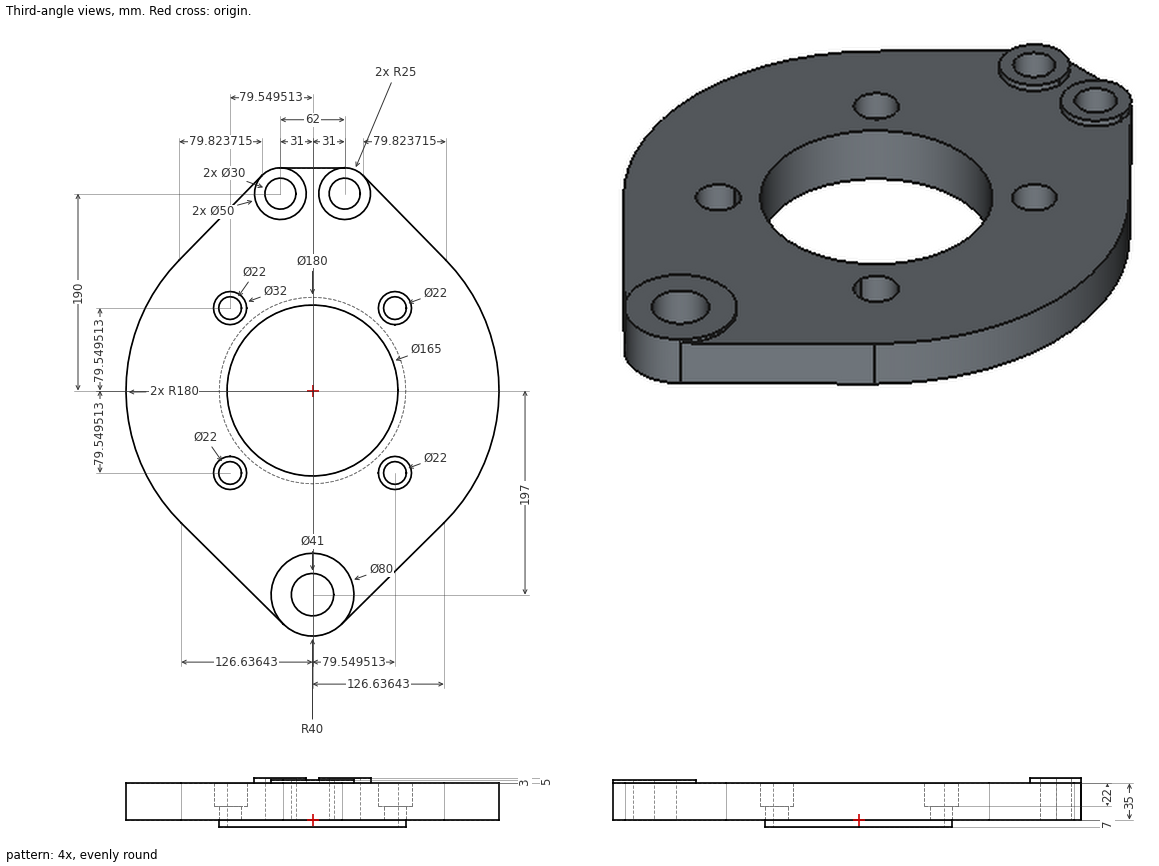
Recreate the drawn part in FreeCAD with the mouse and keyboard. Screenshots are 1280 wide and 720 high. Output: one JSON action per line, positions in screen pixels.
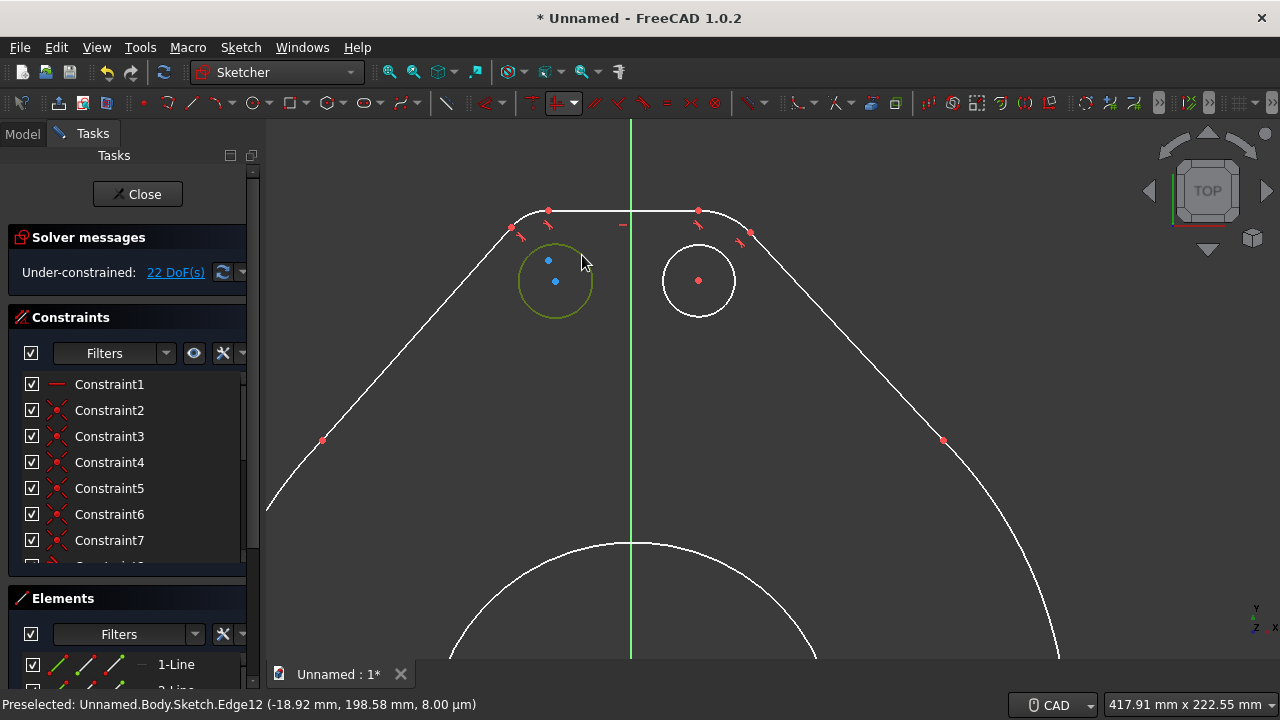
{"action": "left_click", "coordinate": [536, 212]}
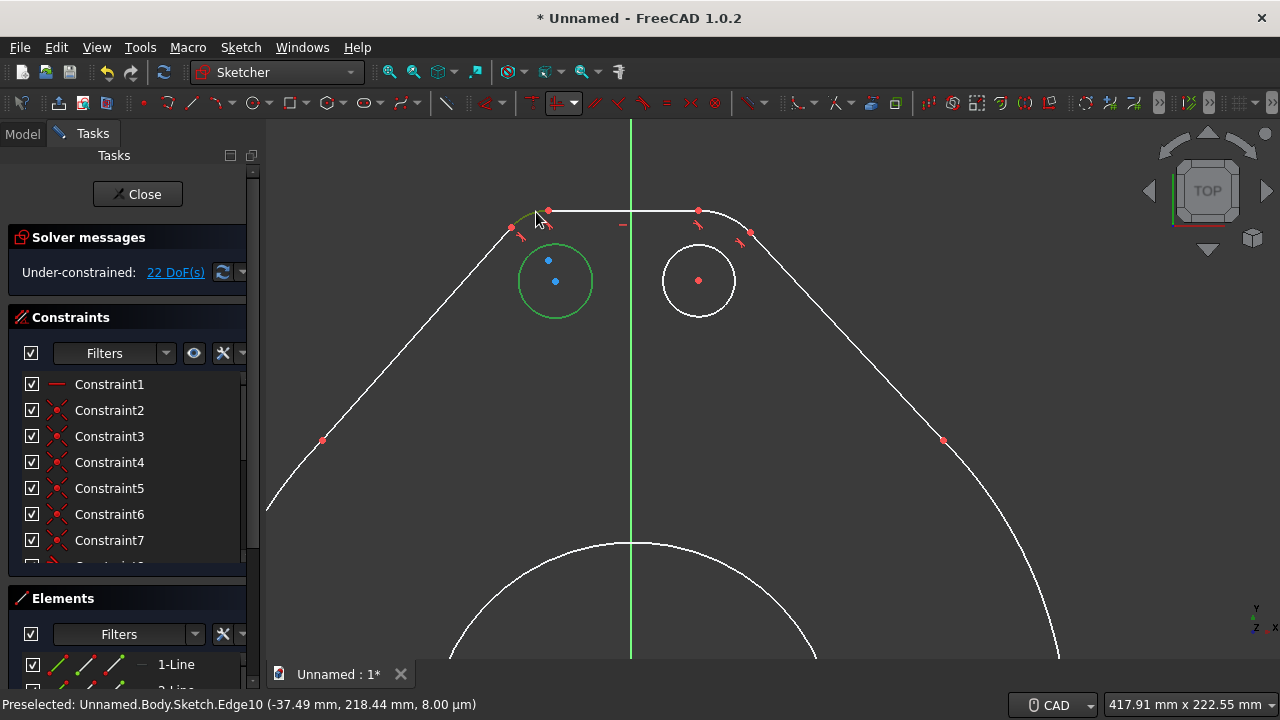
{"action": "key", "text": "c"}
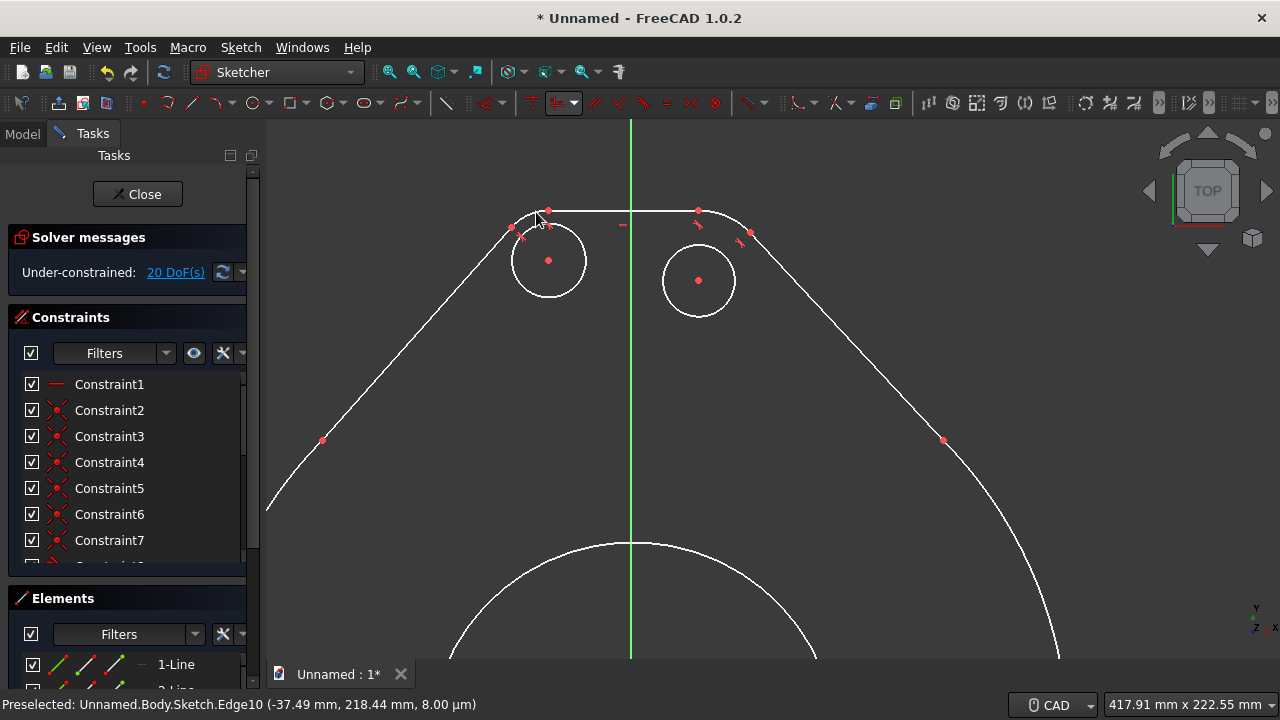
{"action": "scroll", "coordinate": [736, 226], "scroll_direction": "down", "scroll_amount": 6}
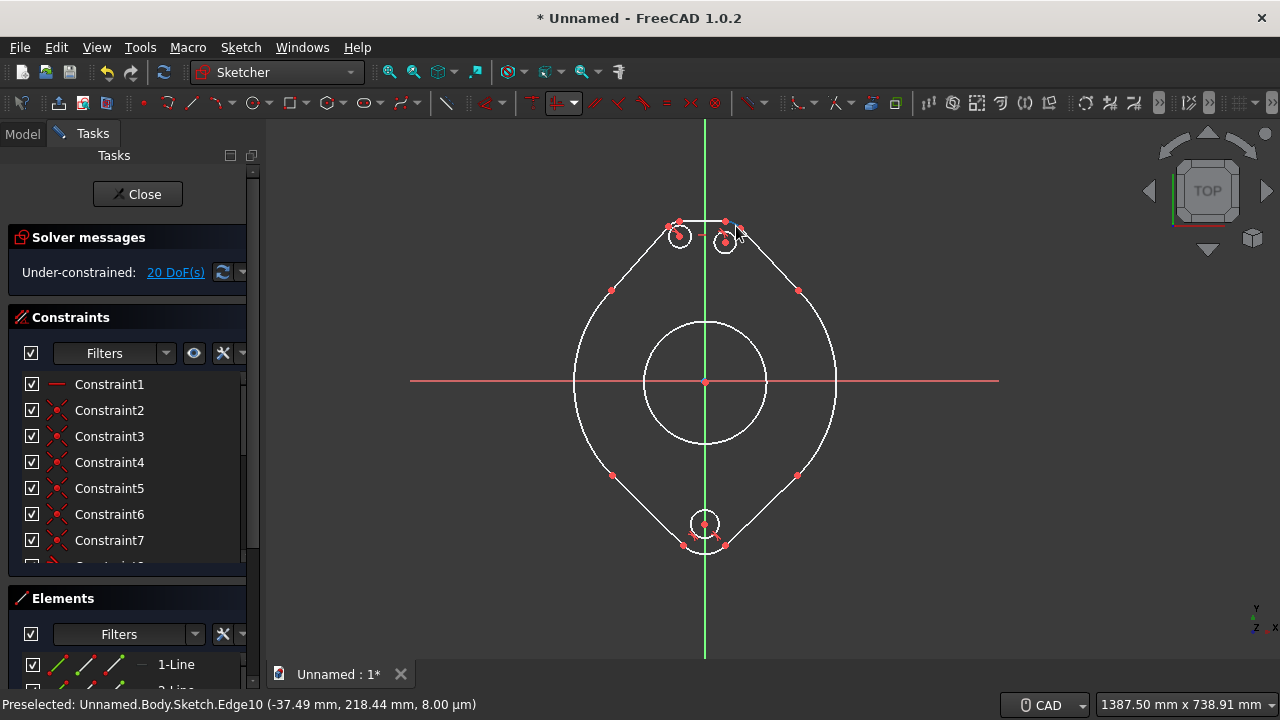
{"action": "scroll", "coordinate": [705, 382], "scroll_direction": "up", "scroll_amount": 7}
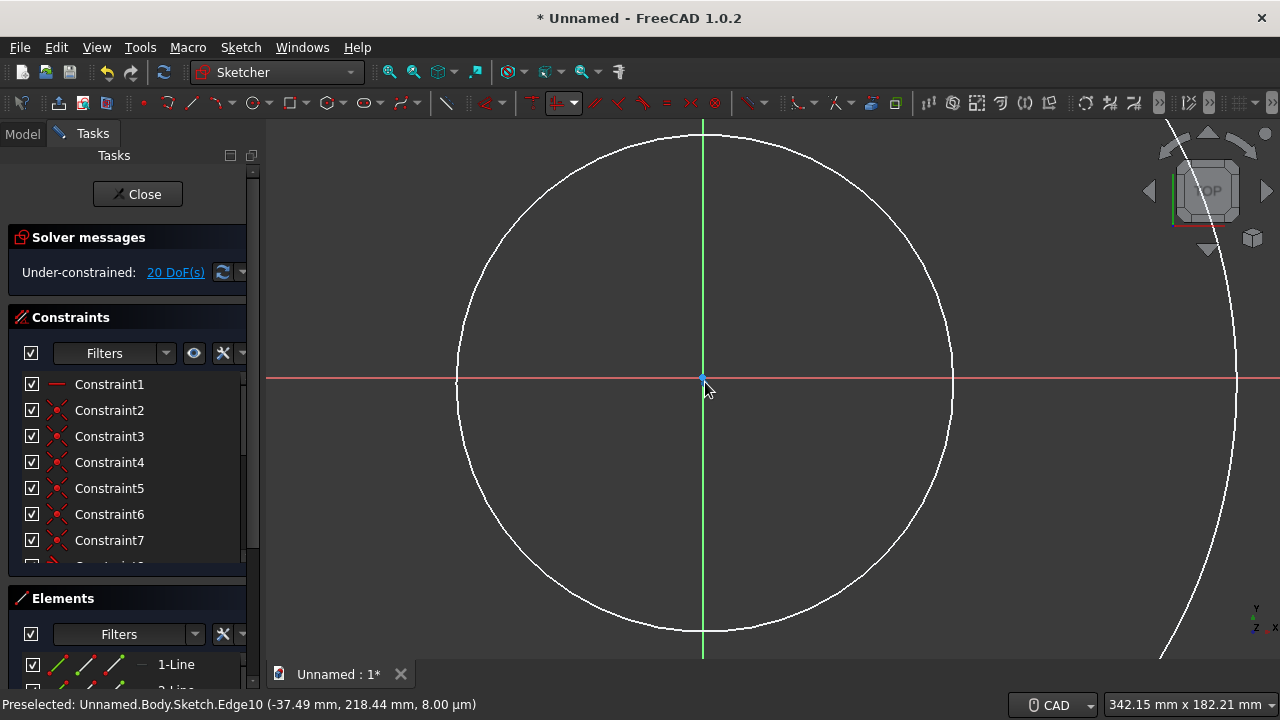
{"action": "left_click_drag", "start_coordinate": [693, 368], "coordinate": [715, 393]}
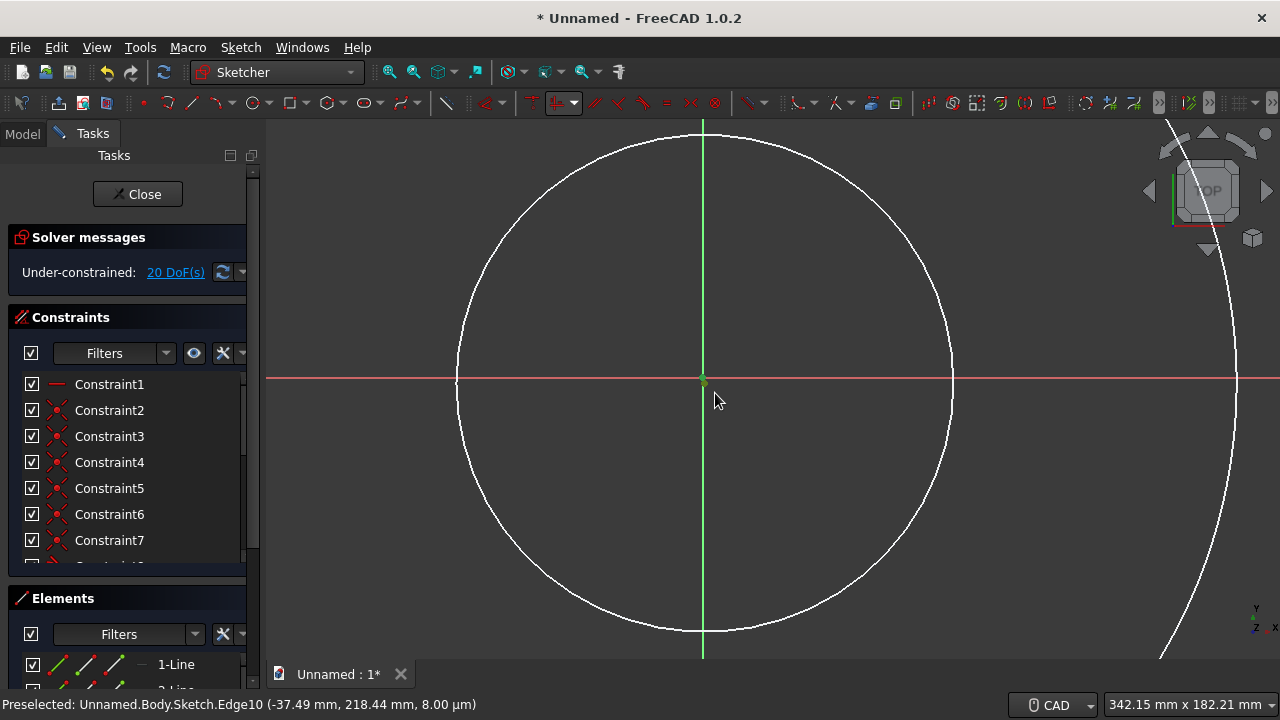
{"action": "key", "text": "c"}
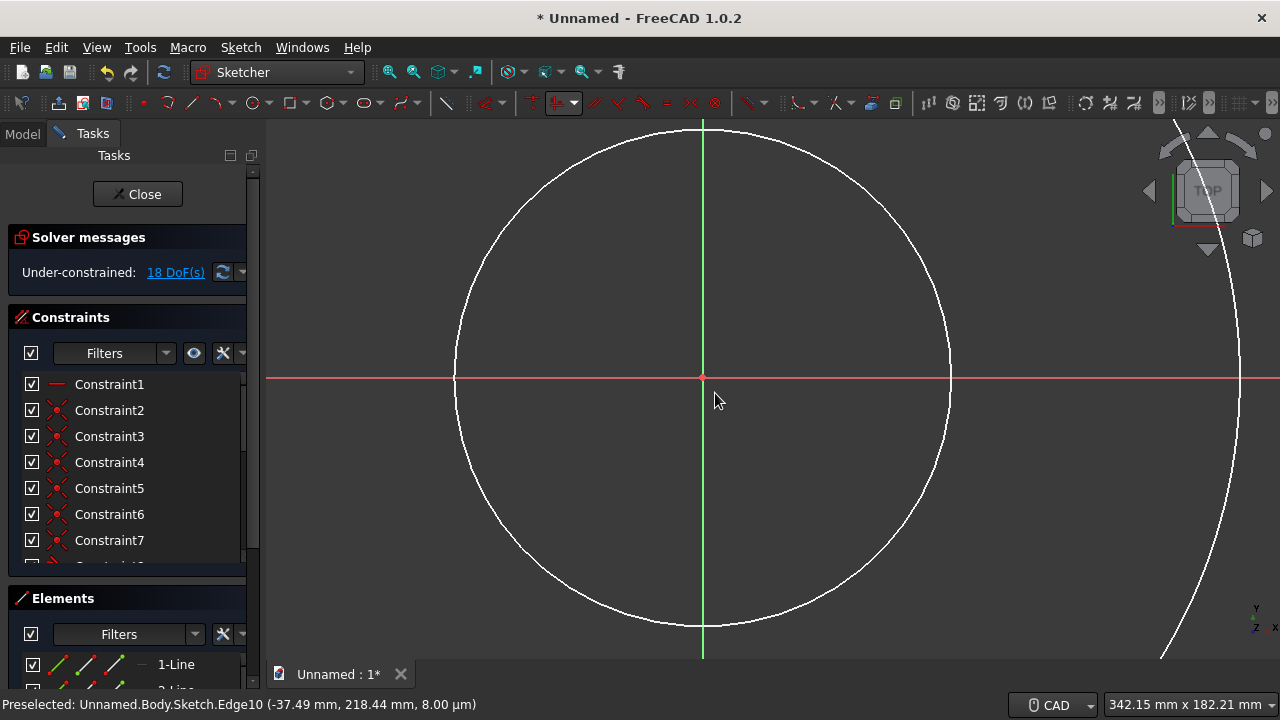
{"action": "scroll", "coordinate": [705, 382], "scroll_direction": "down", "scroll_amount": 7}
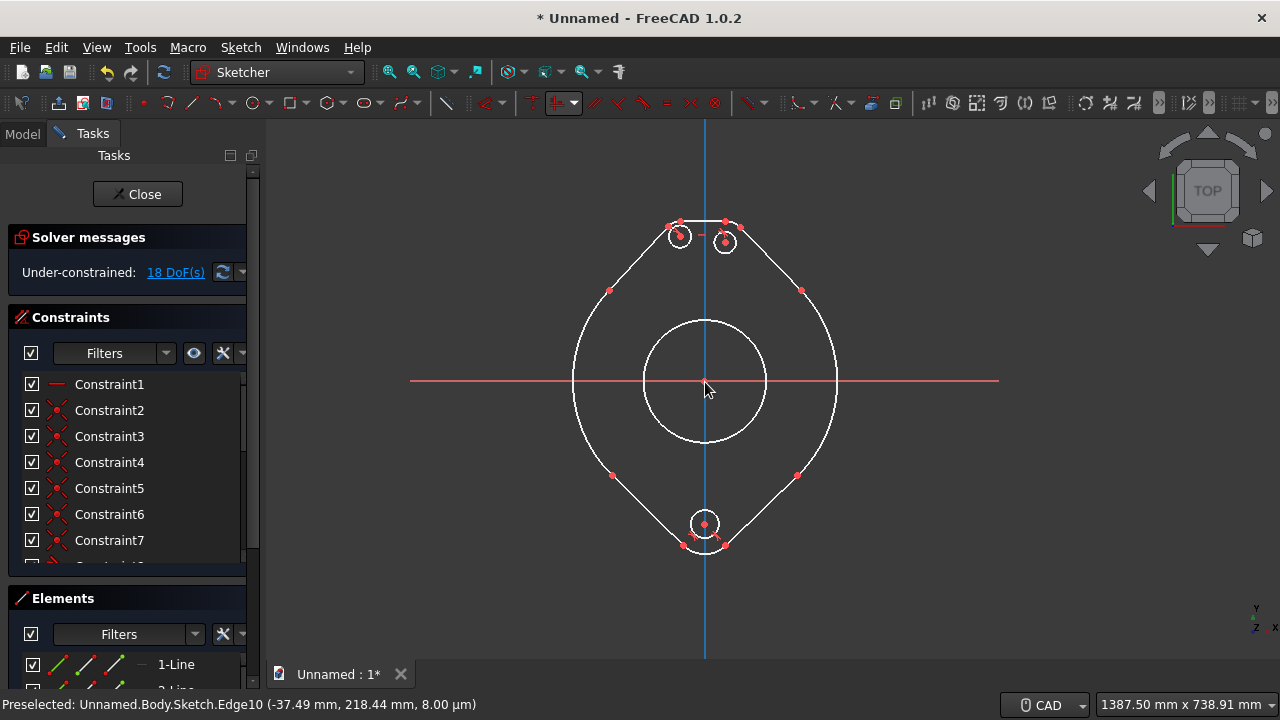
{"action": "left_click", "coordinate": [578, 344]}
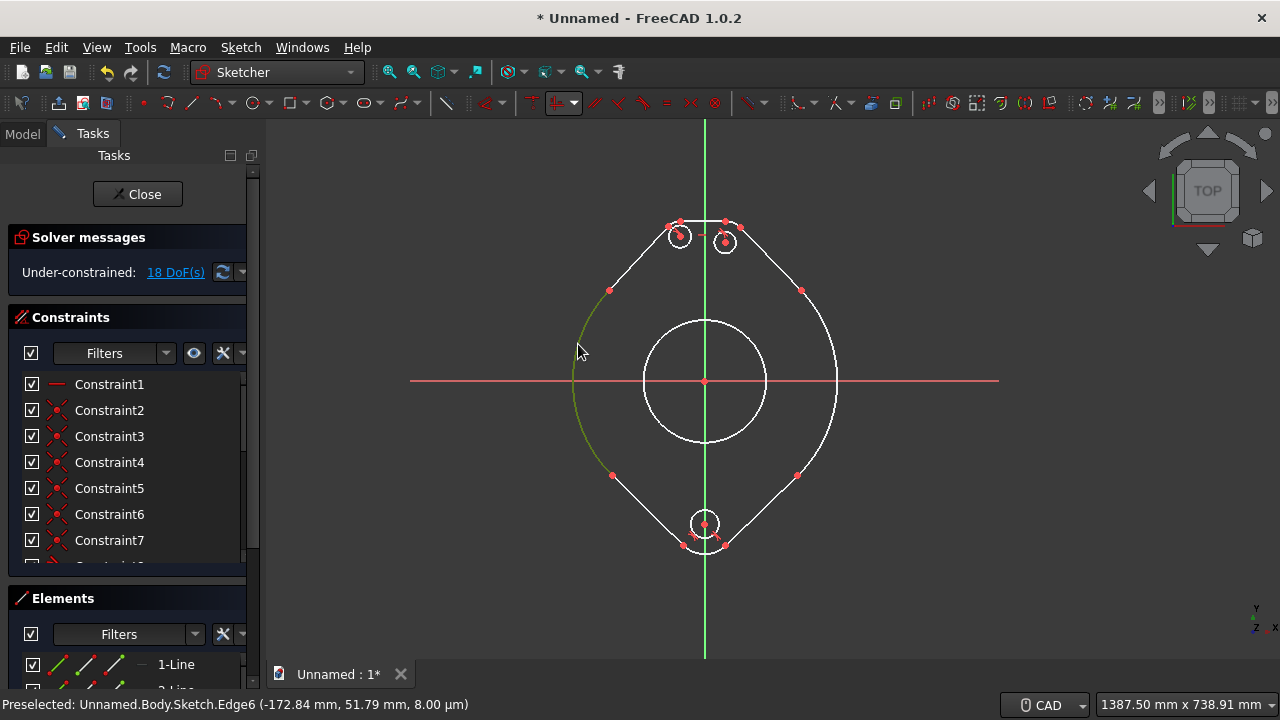
{"action": "left_click", "coordinate": [830, 424]}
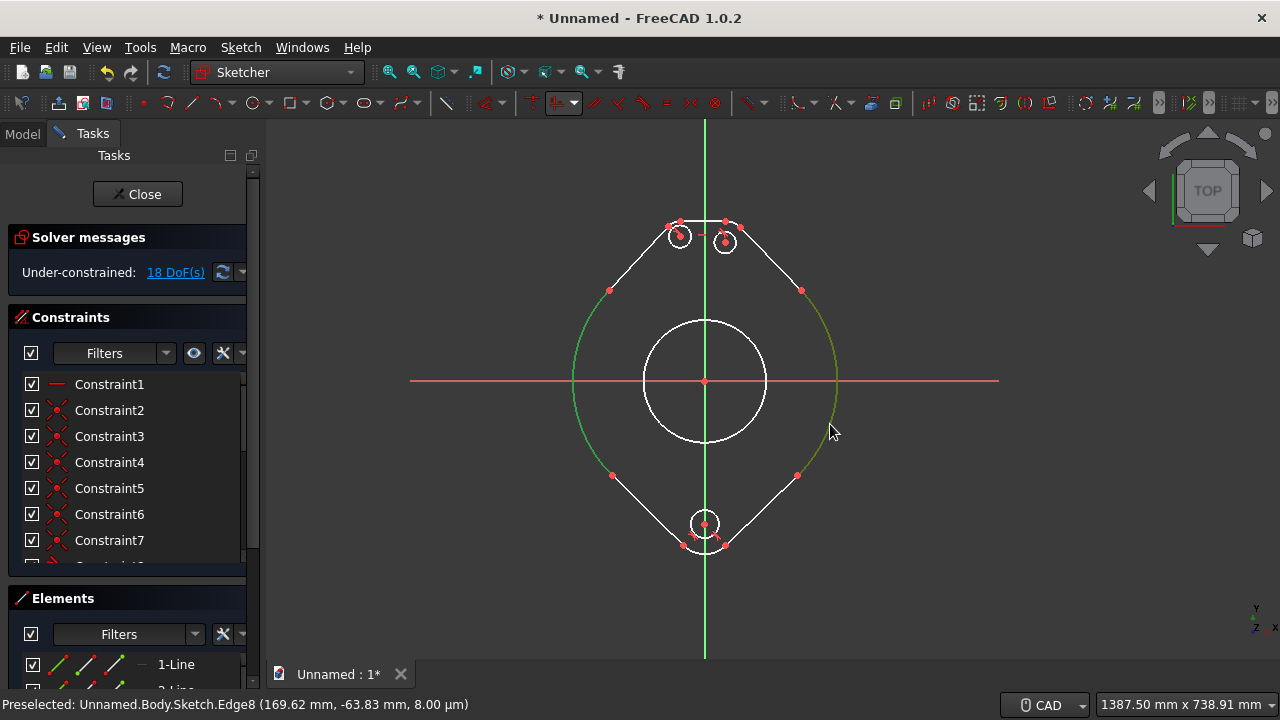
{"action": "key", "text": "e"}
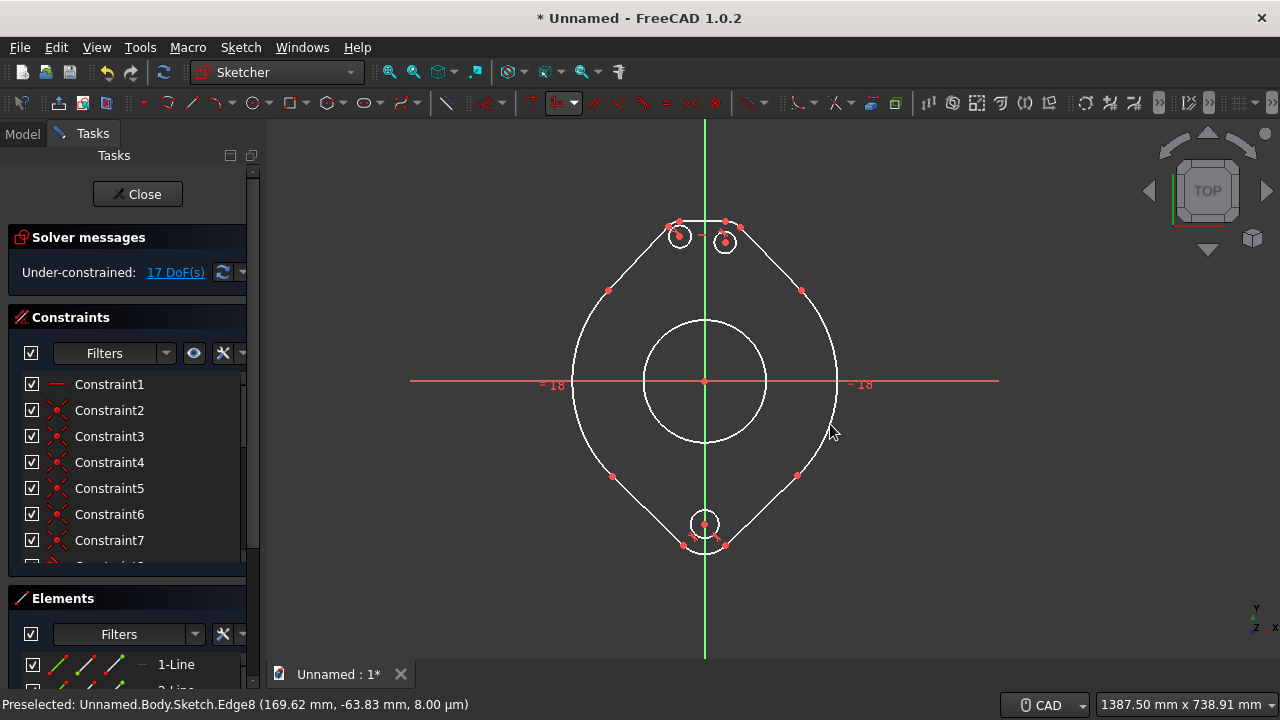
{"action": "scroll", "coordinate": [734, 223], "scroll_direction": "up", "scroll_amount": 3}